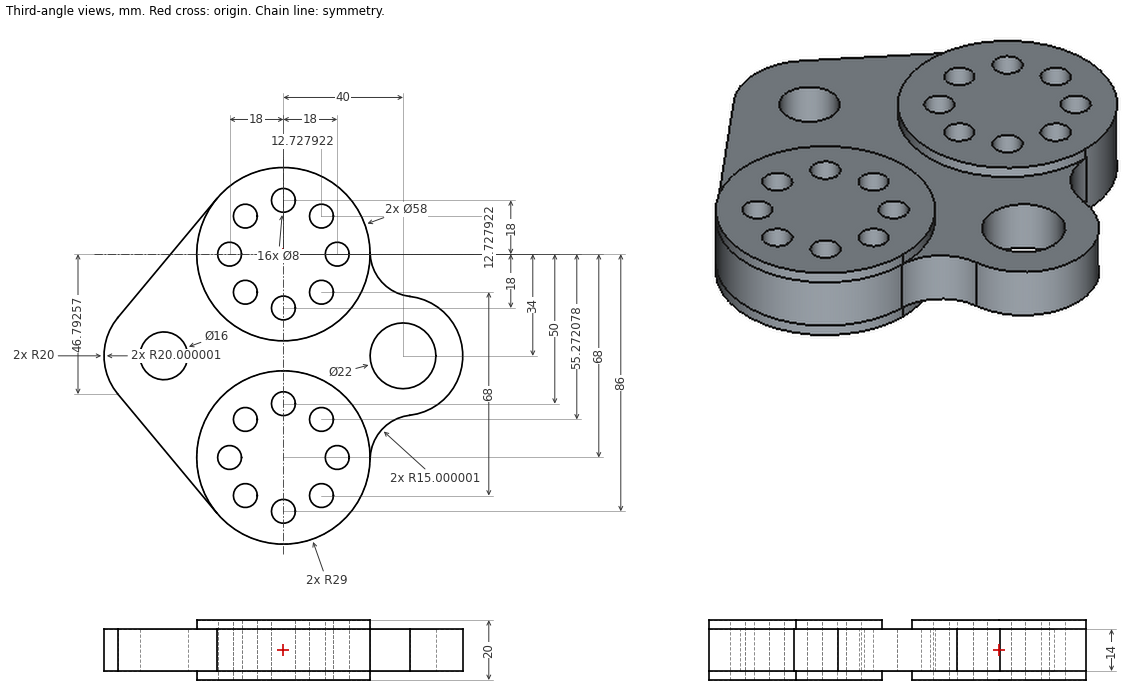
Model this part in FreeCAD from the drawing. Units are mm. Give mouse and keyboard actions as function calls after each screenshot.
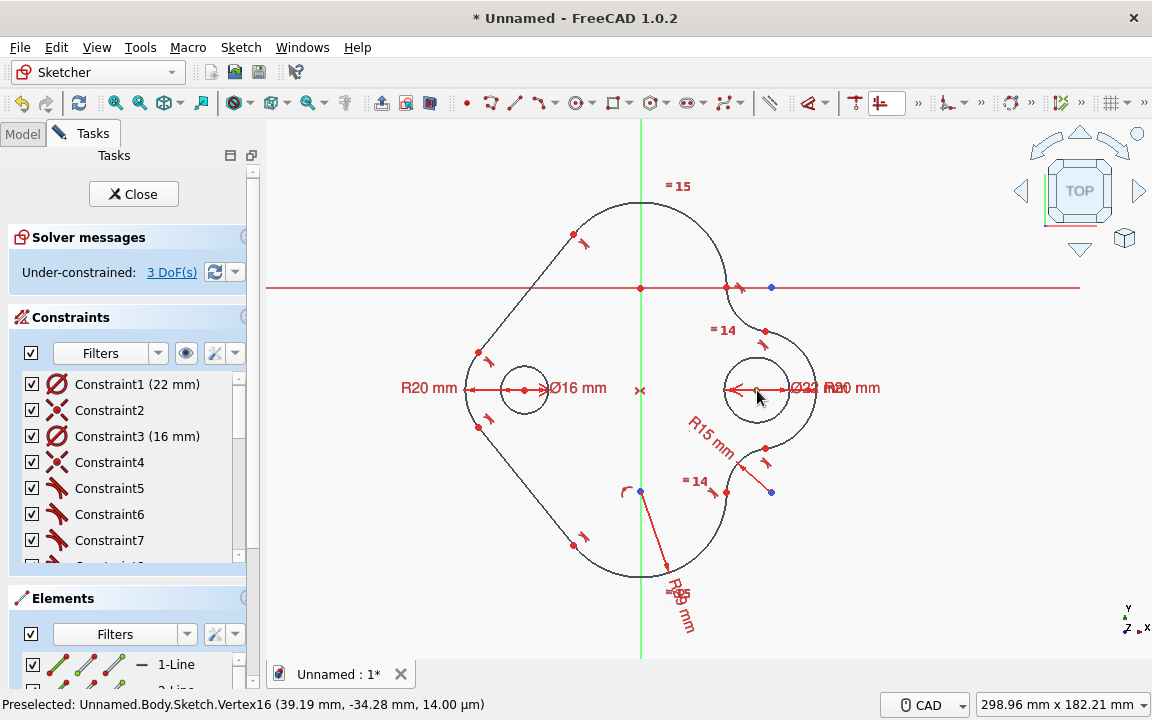
key(l)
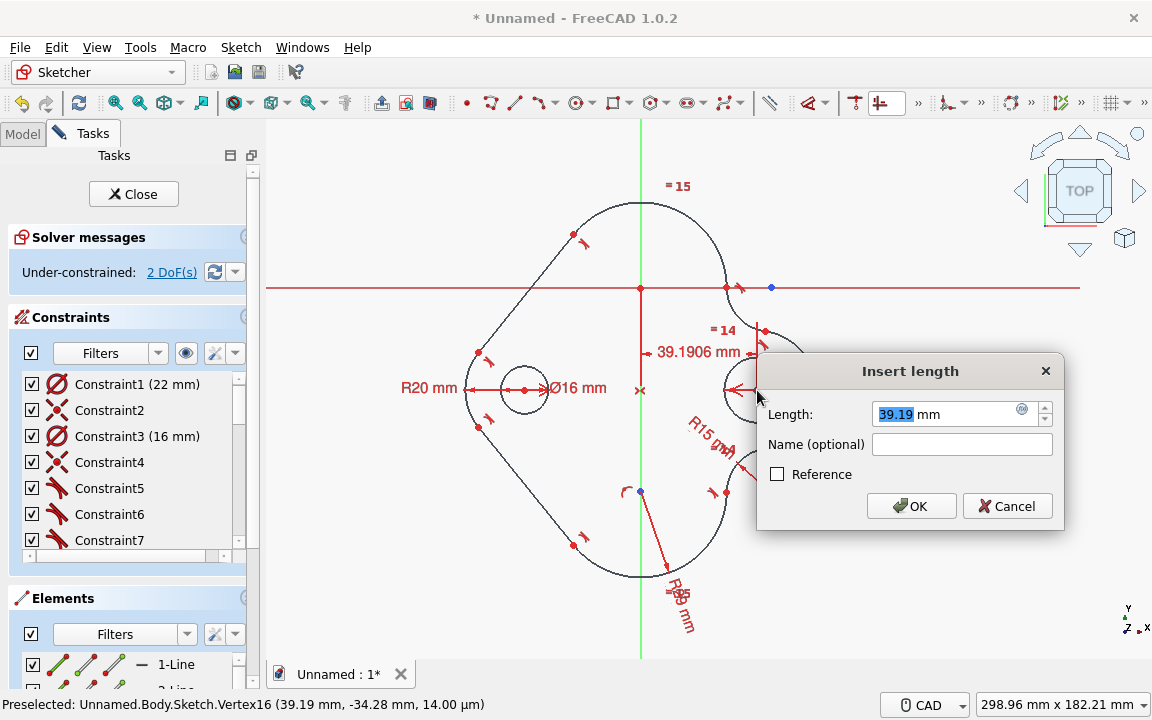
text(40)
key(Return)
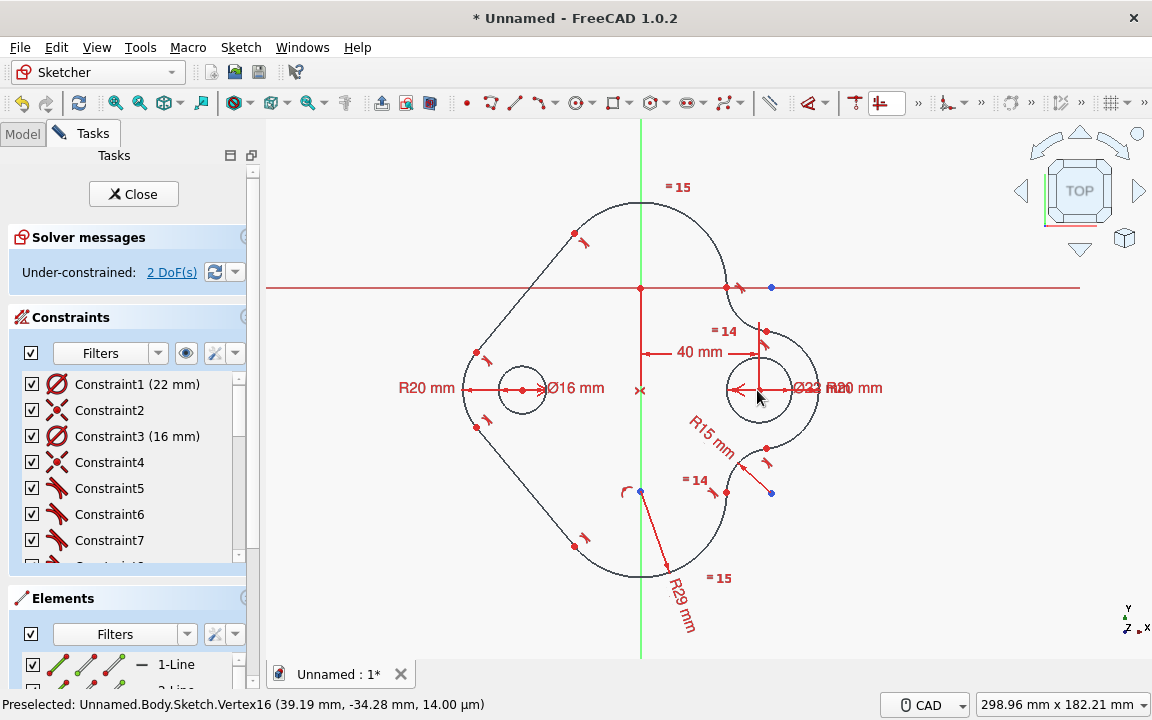
click(759, 390)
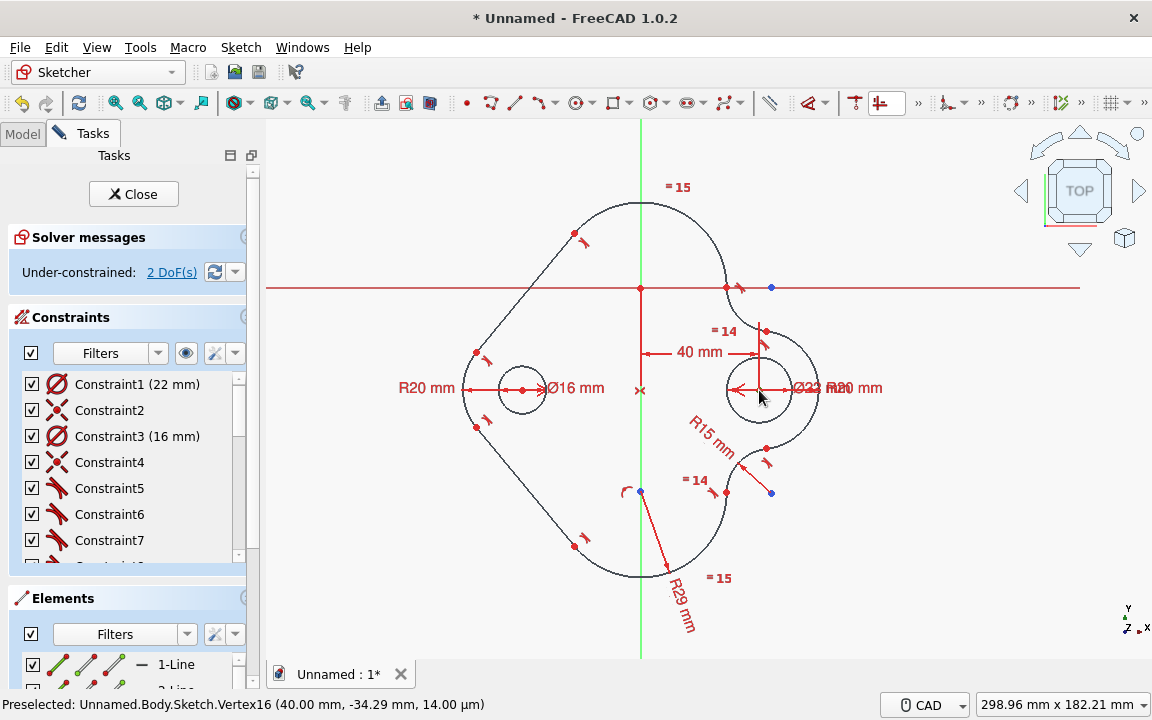
key(i)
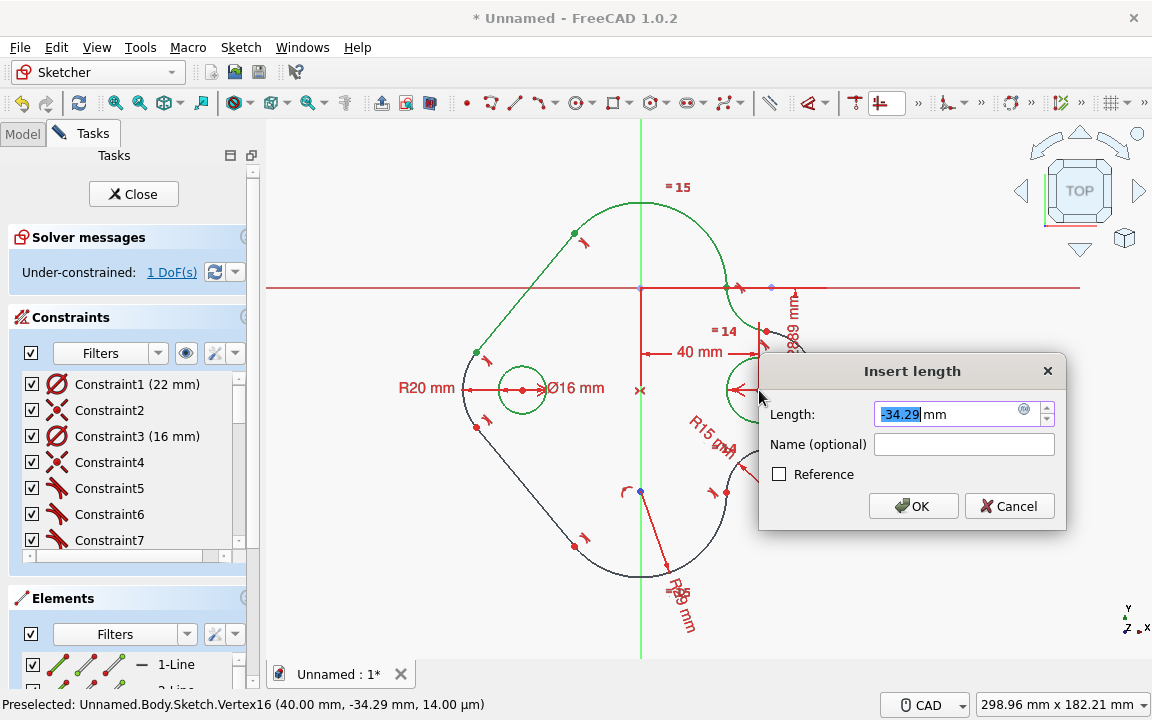
text(-34)
key(Return)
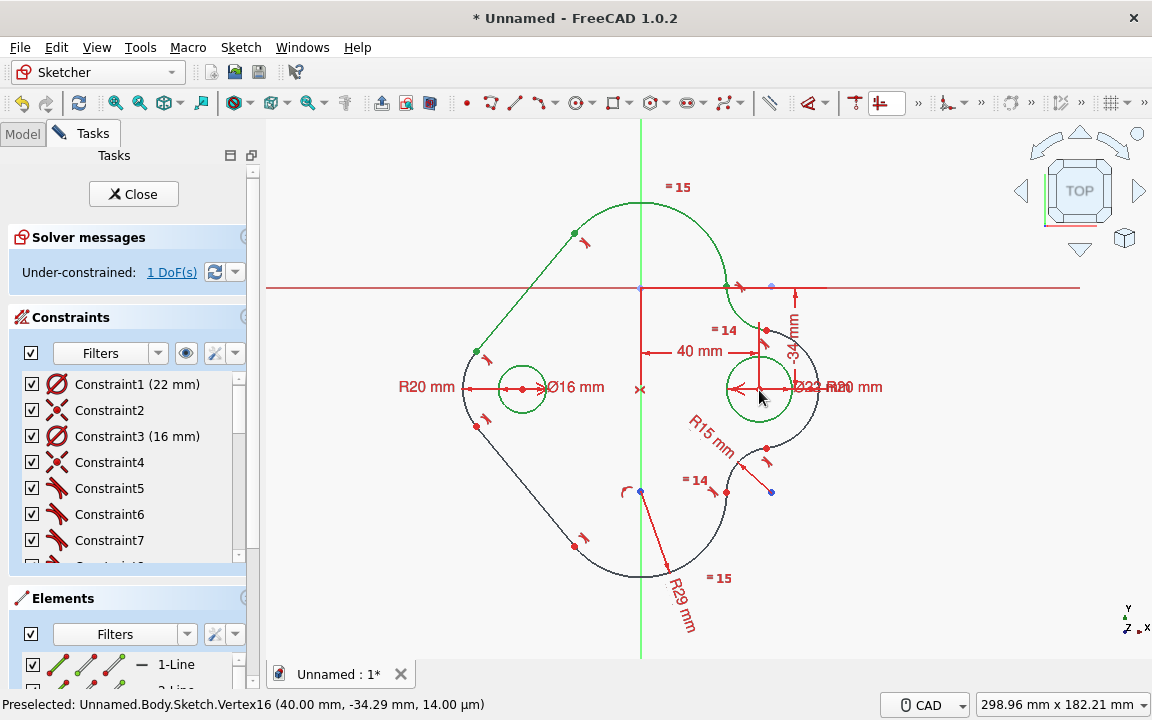
click(477, 427)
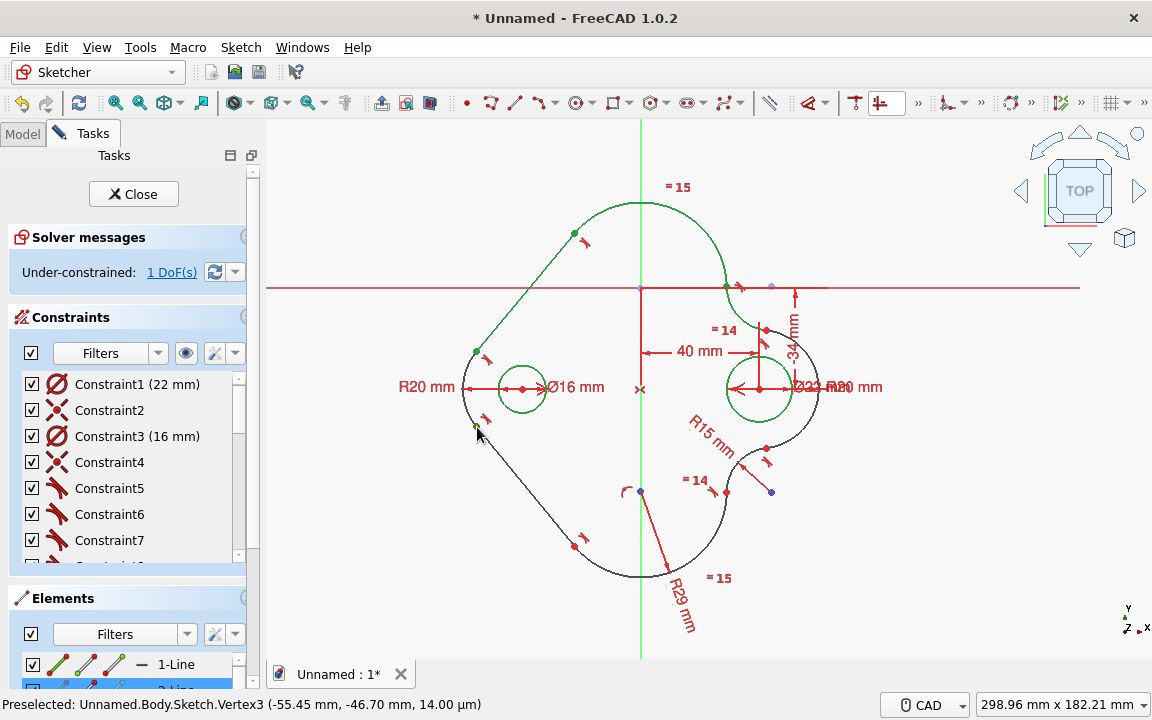
key(i)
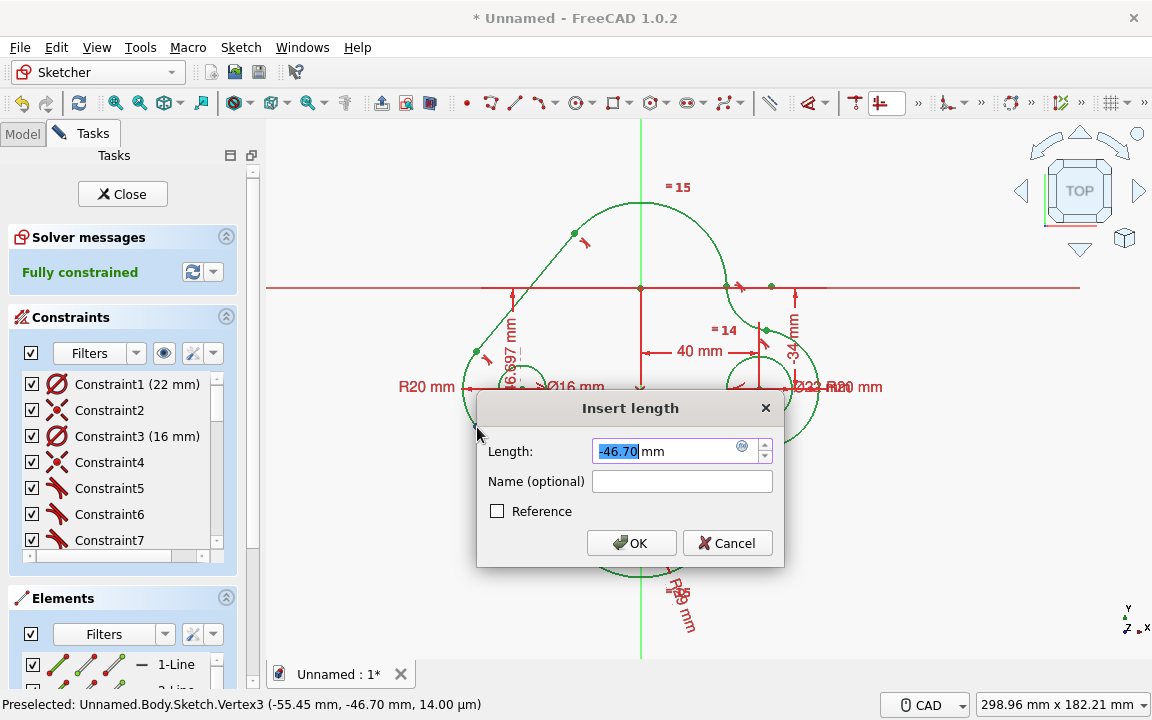
text(-46.79257)
key(Return)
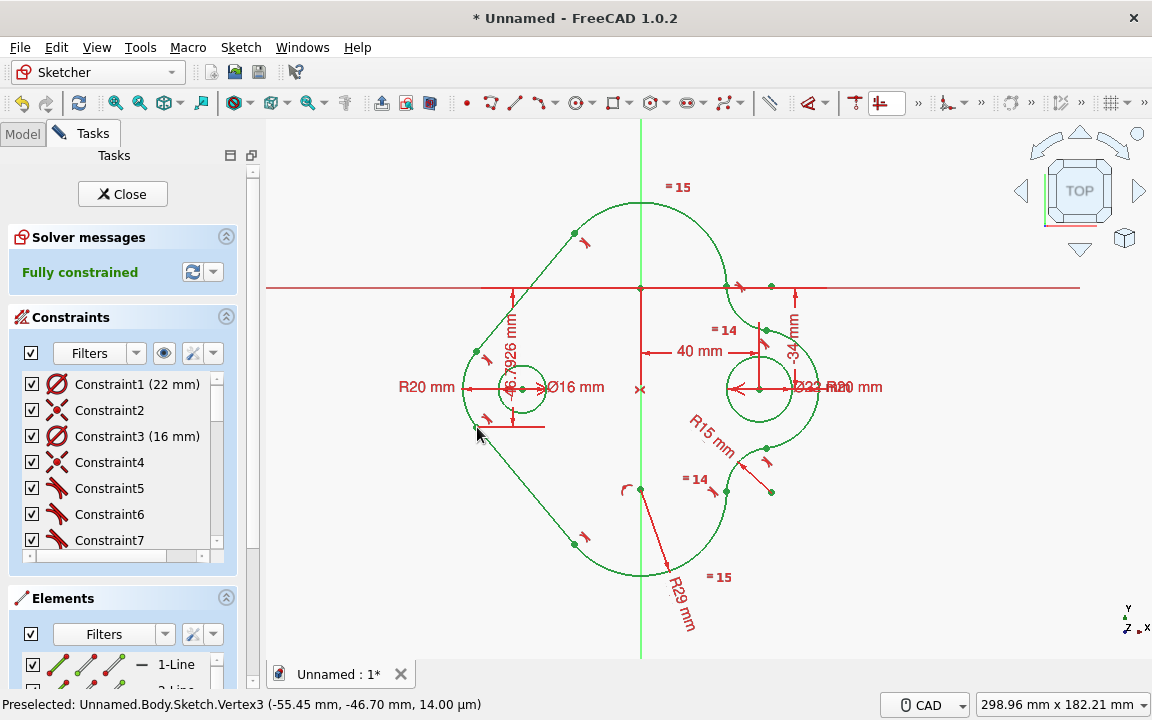
click(123, 194)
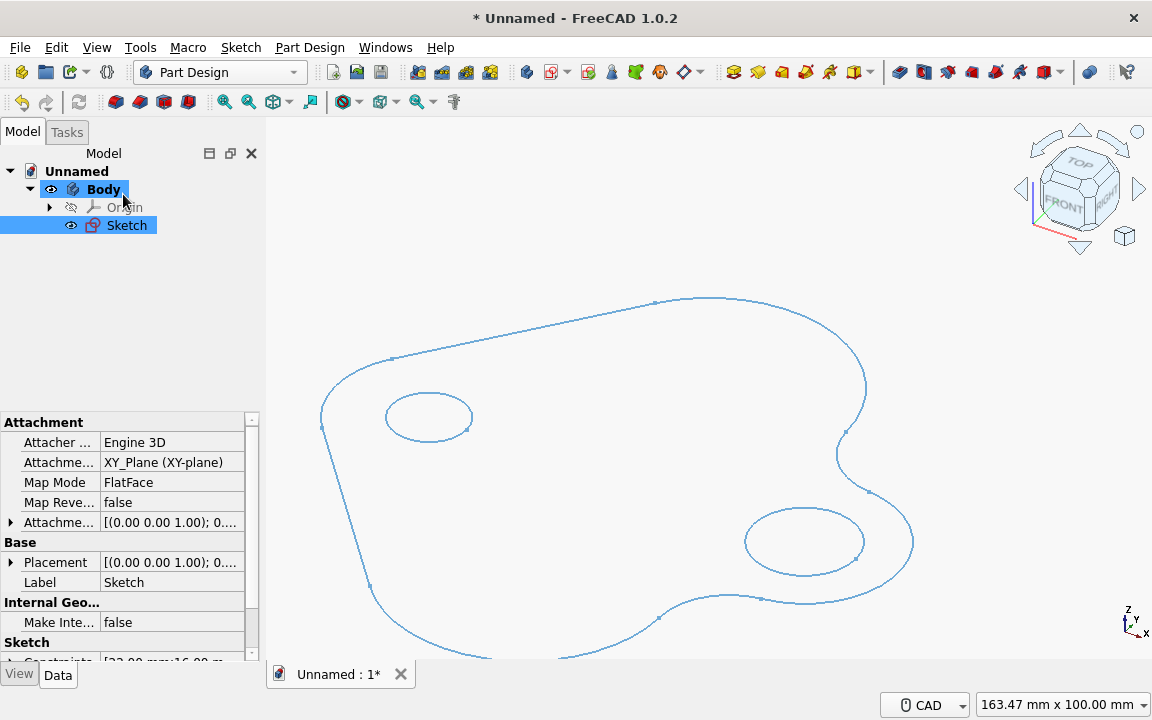
click(734, 72)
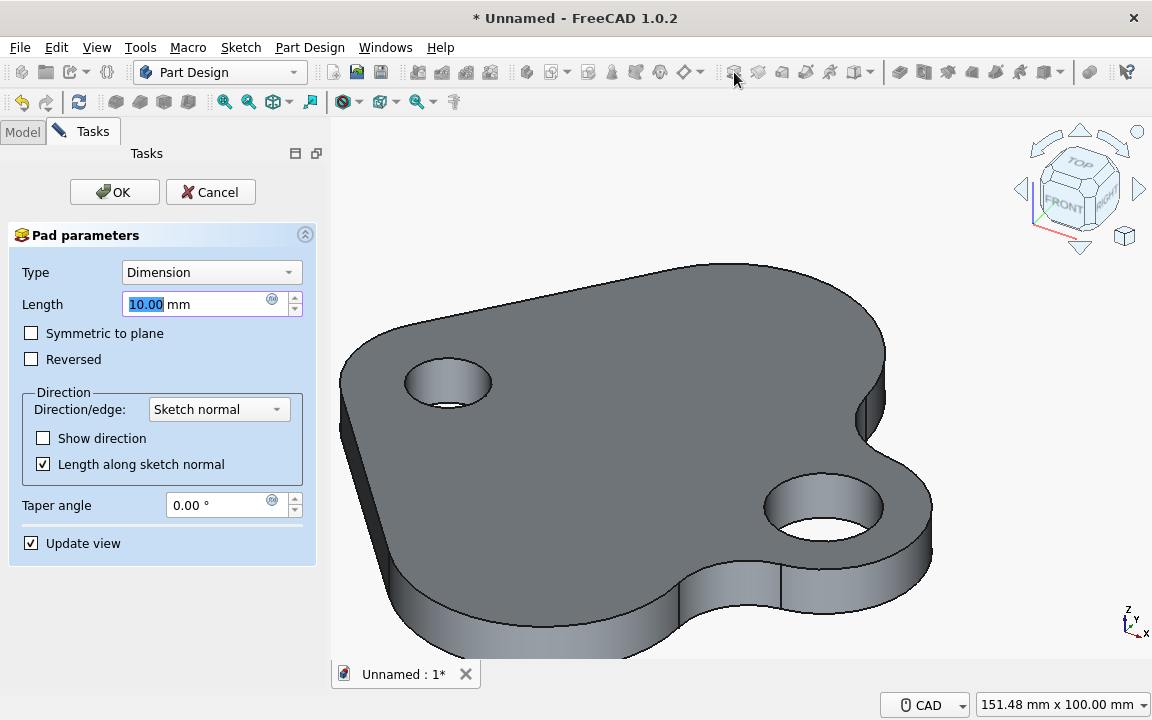
text(14)
key(Tab)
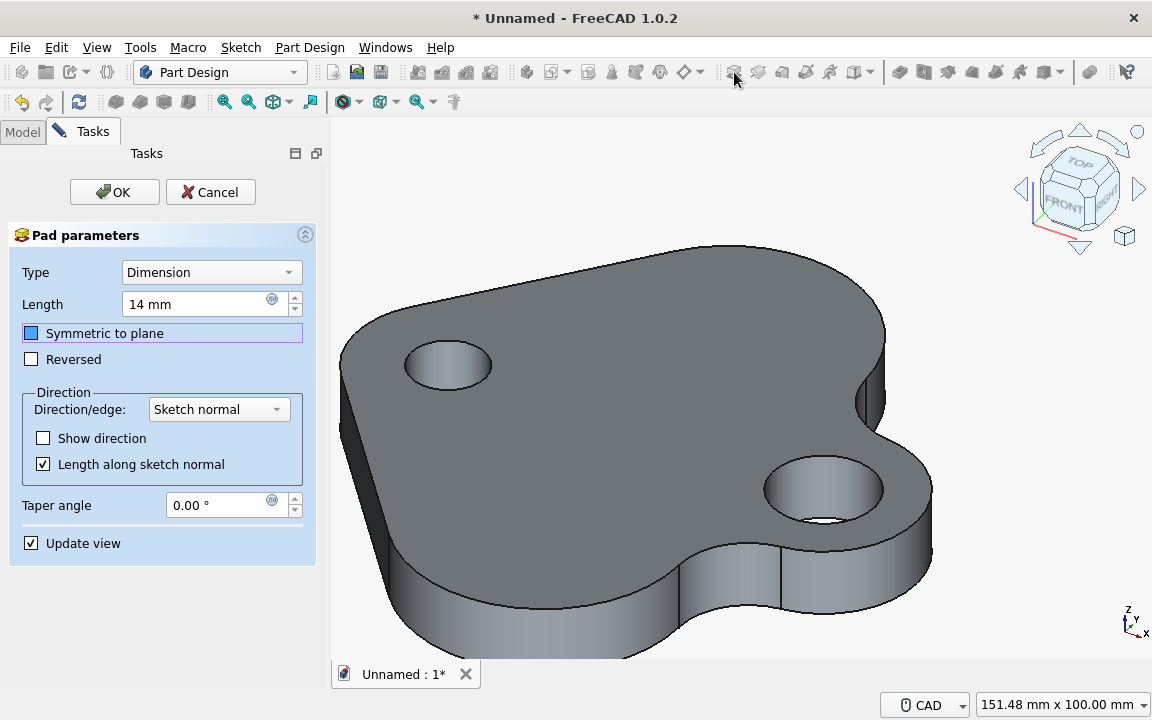
click(30, 333)